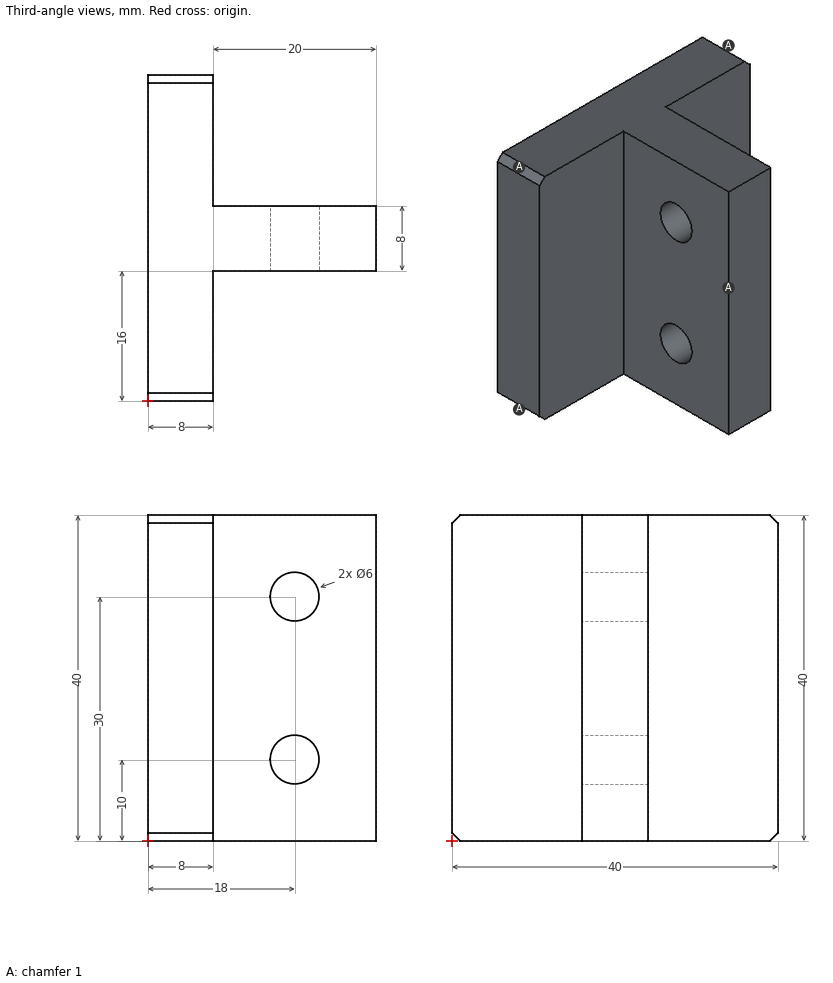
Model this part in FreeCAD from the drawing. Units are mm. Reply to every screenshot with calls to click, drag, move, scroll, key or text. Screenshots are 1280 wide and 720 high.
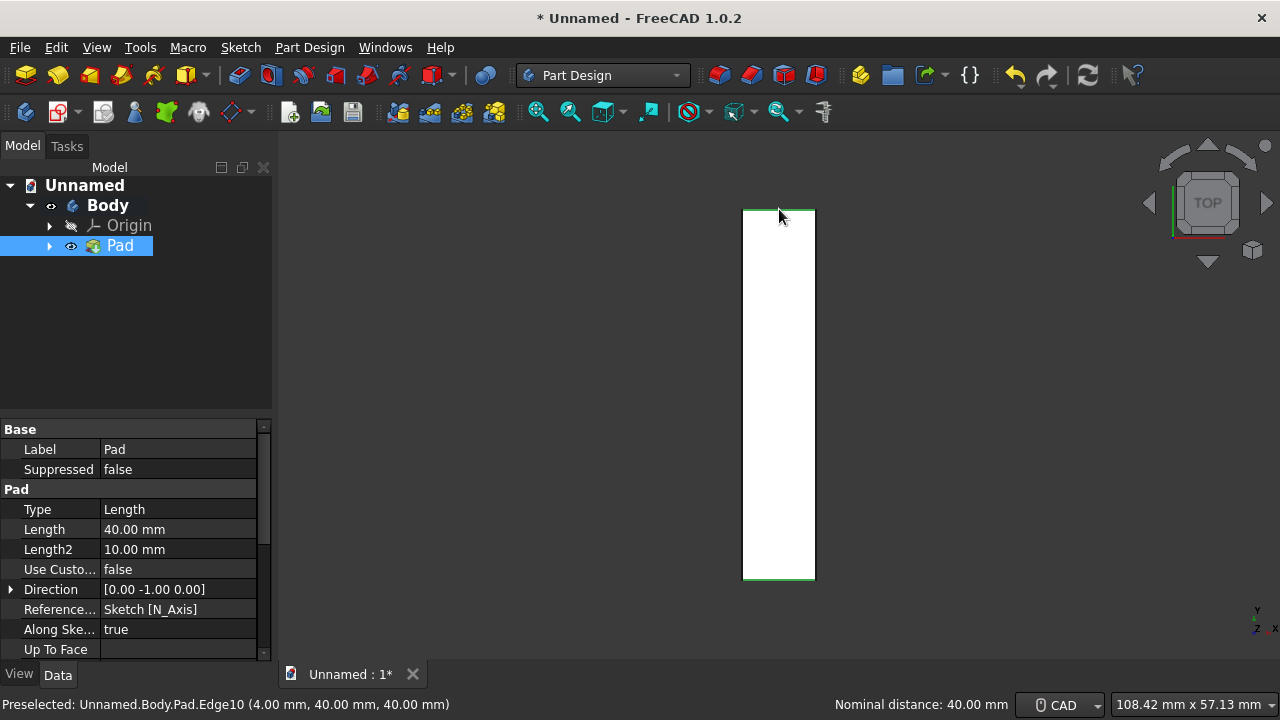
key(1)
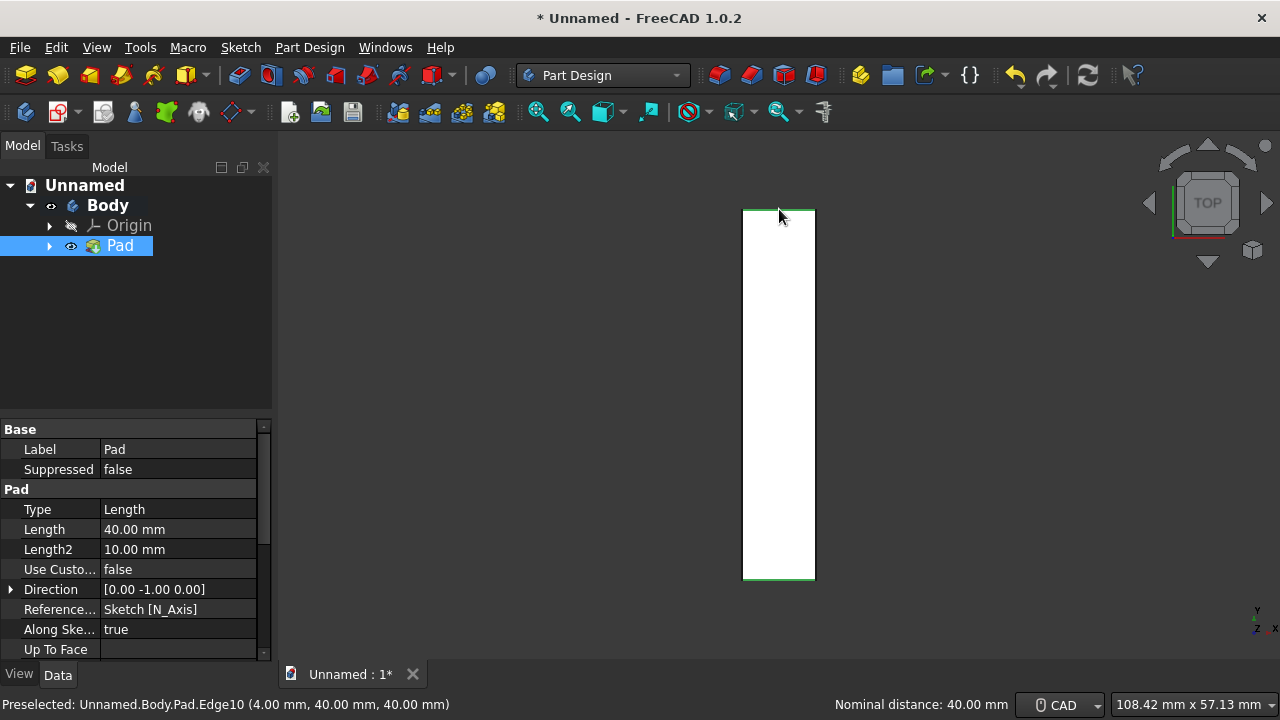
key(3)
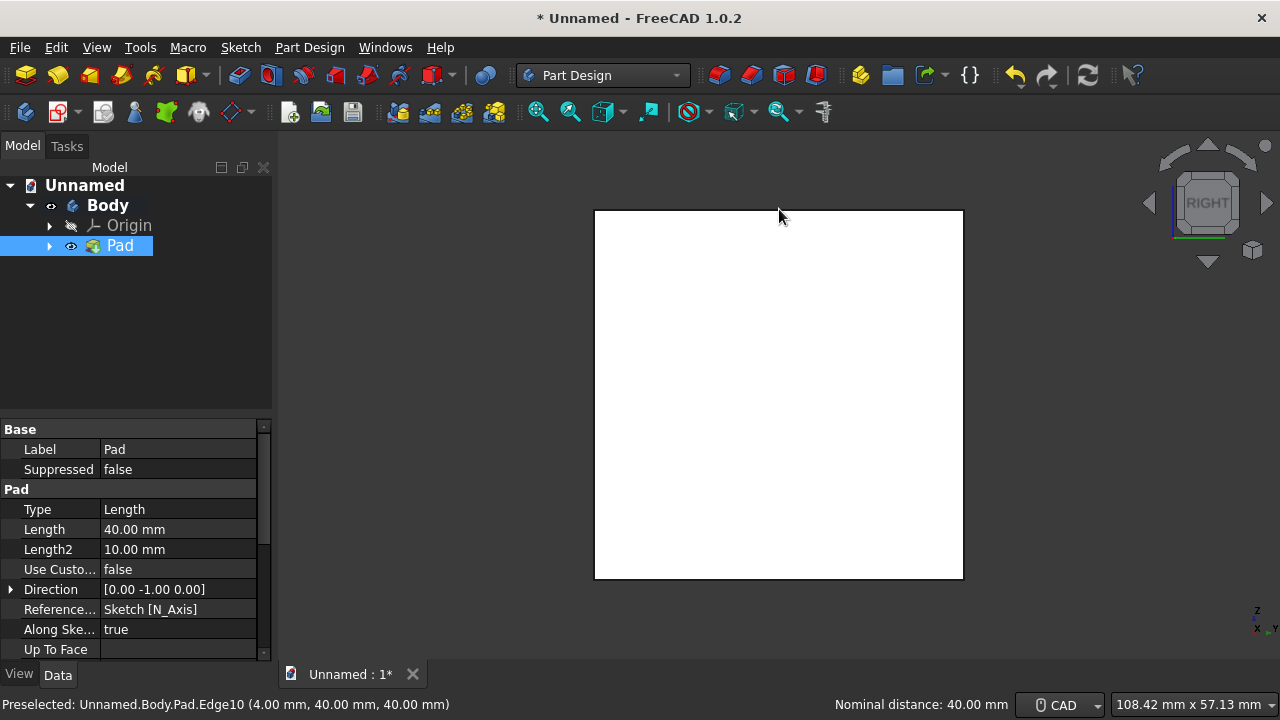
key(5)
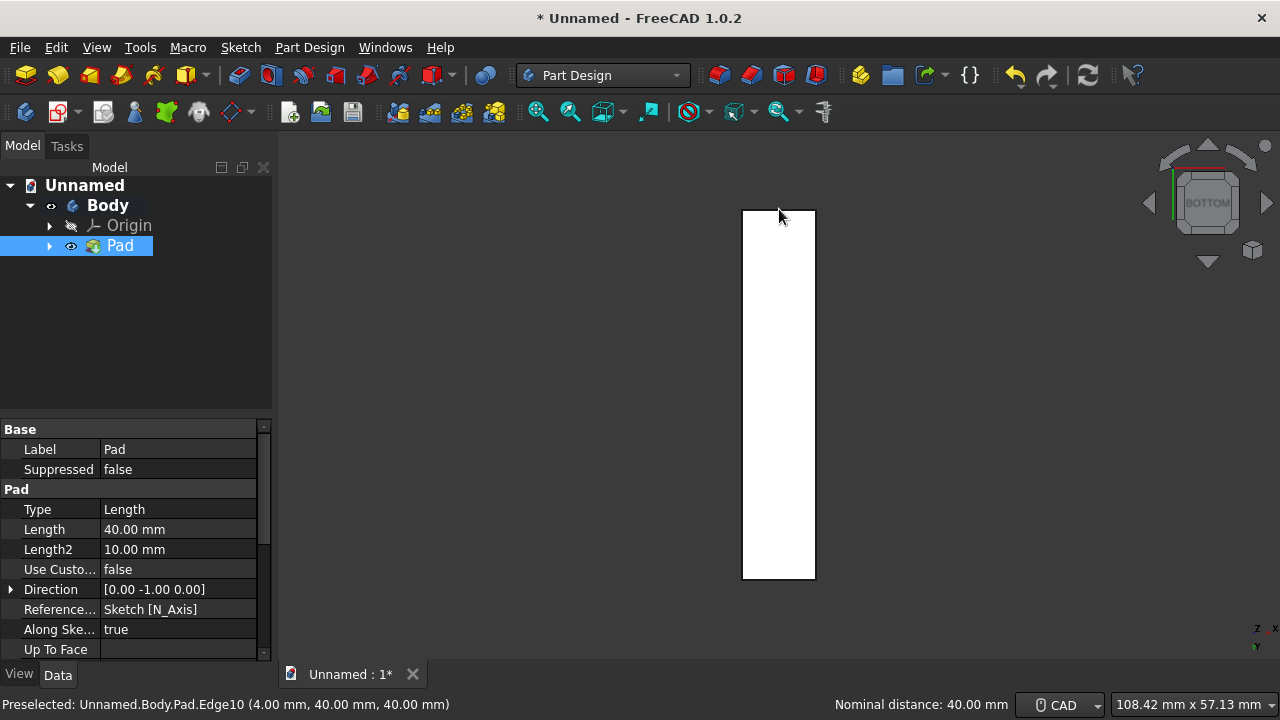
click(779, 209, ctrl)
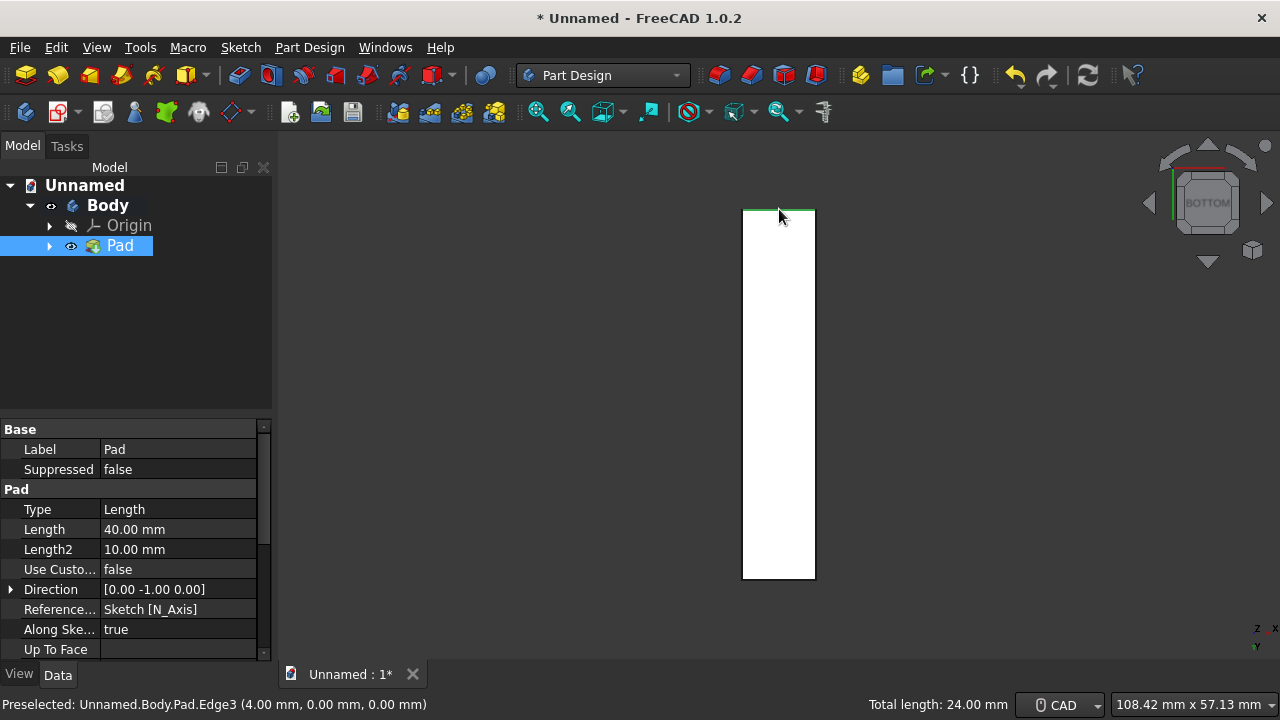
key(4)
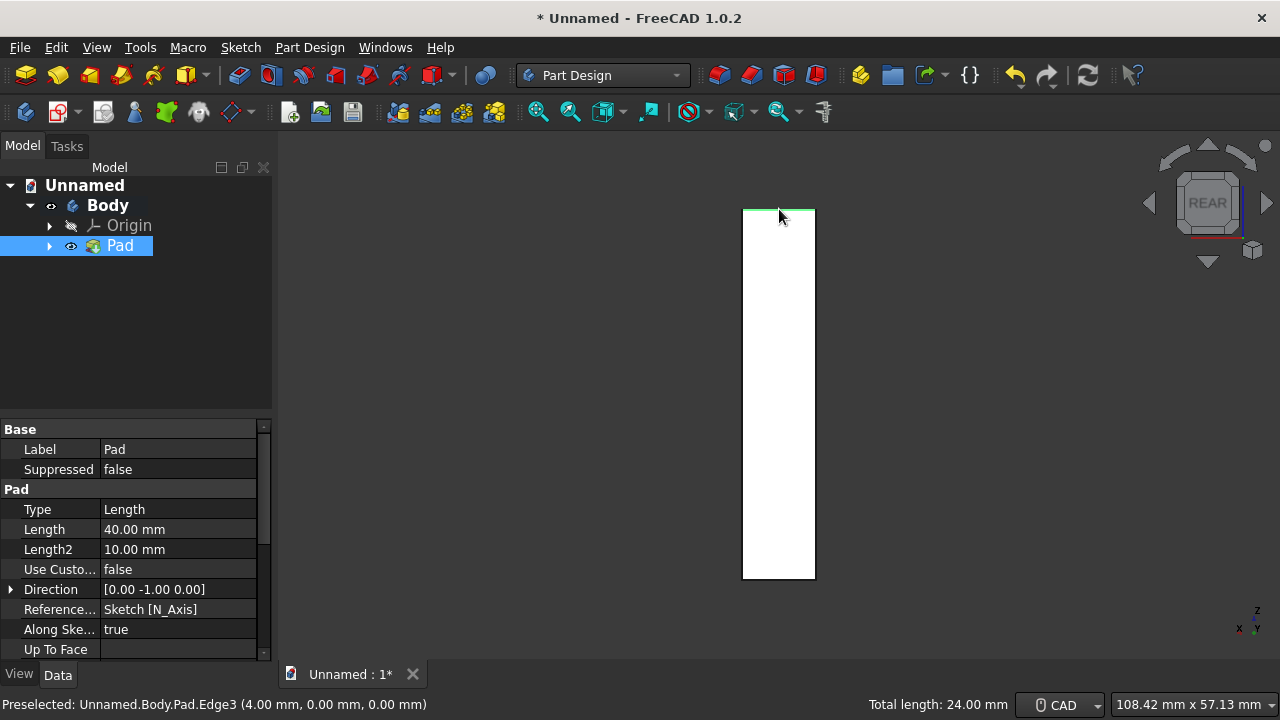
click(779, 579, ctrl)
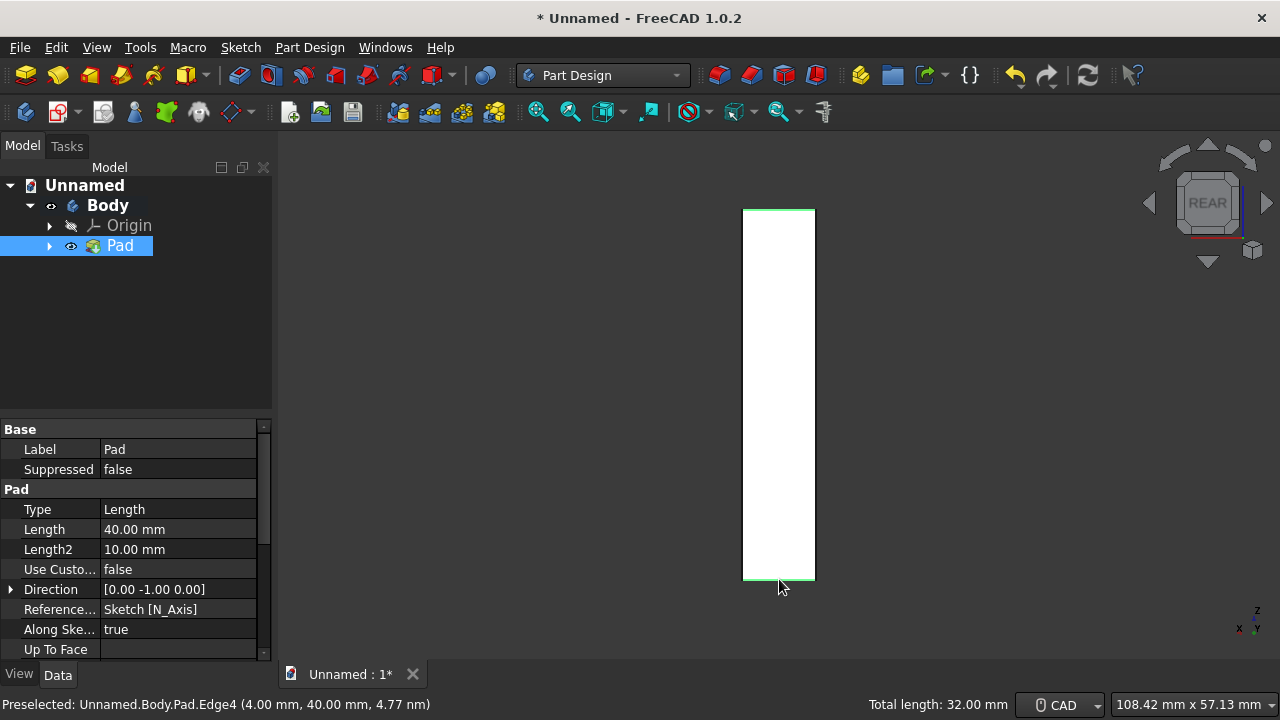
click(752, 76)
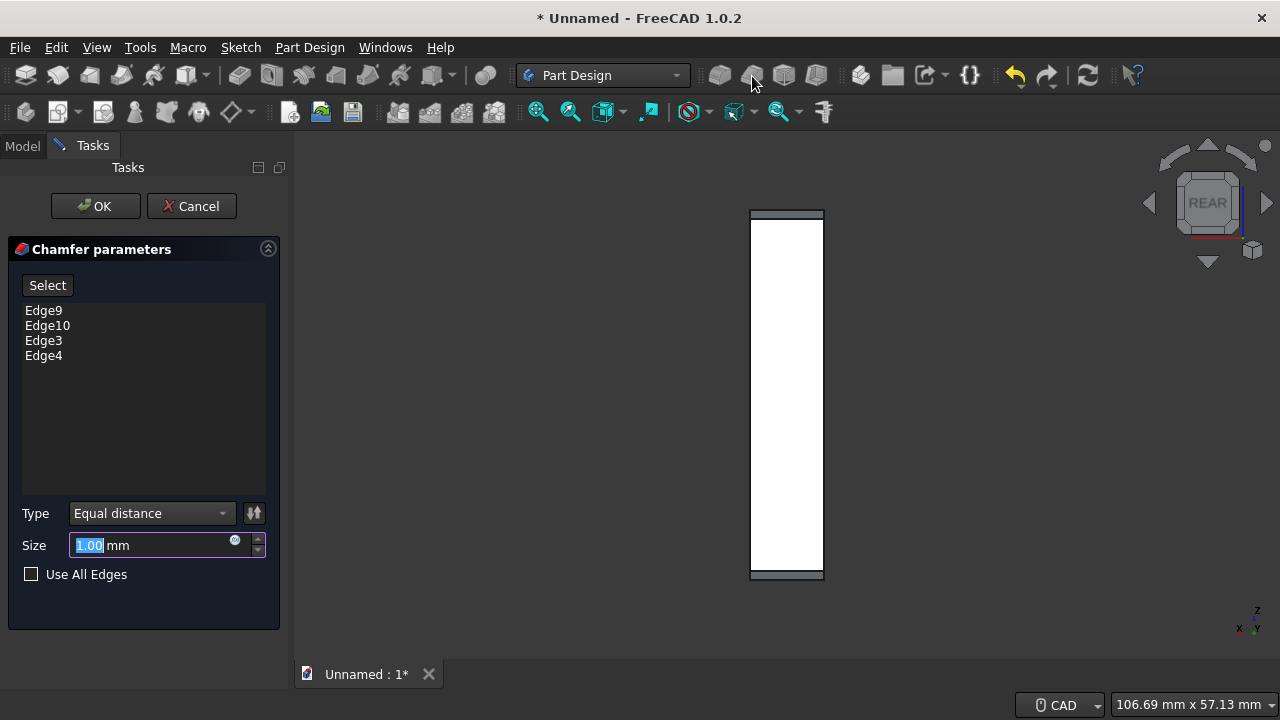
text(1)
key(Tab)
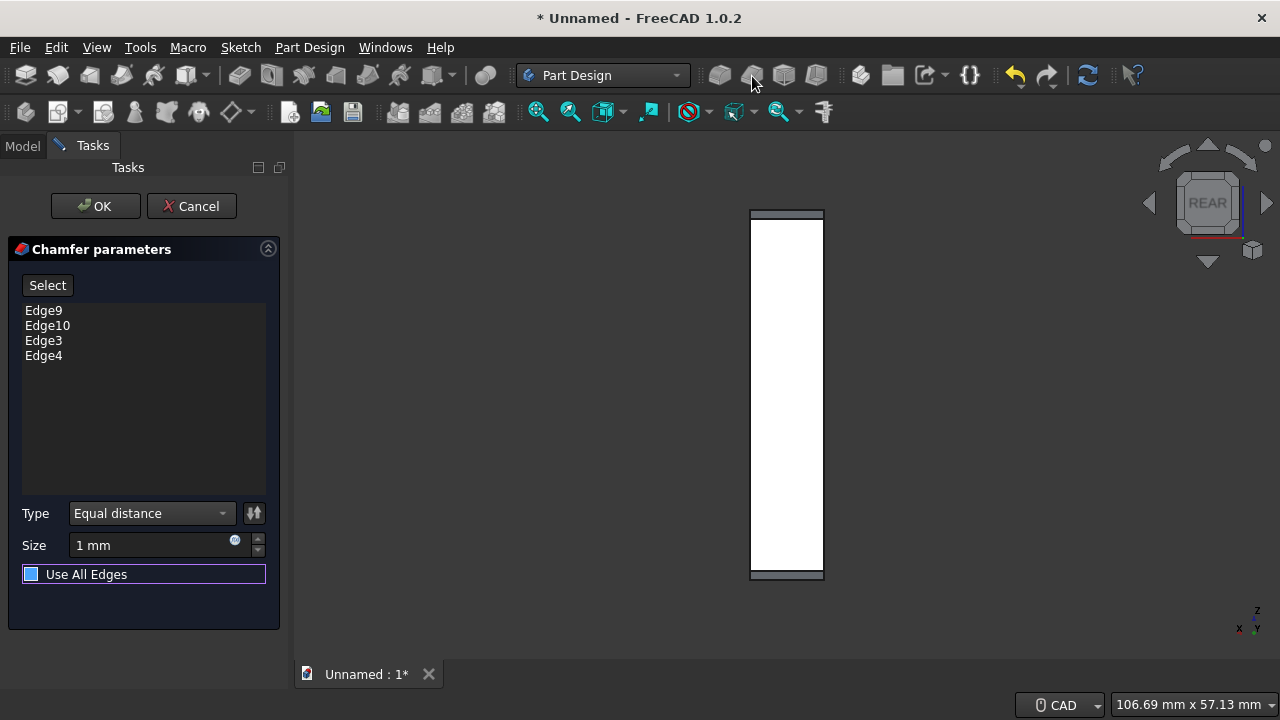
click(96, 206)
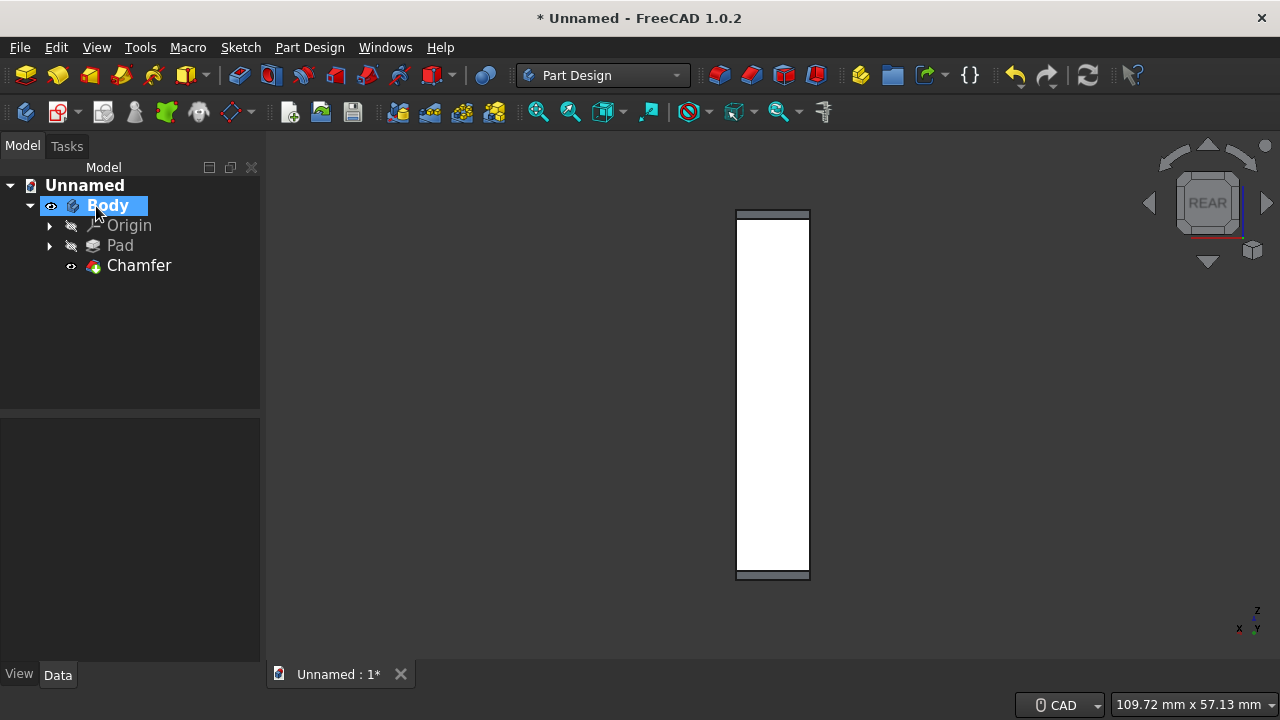
key(0)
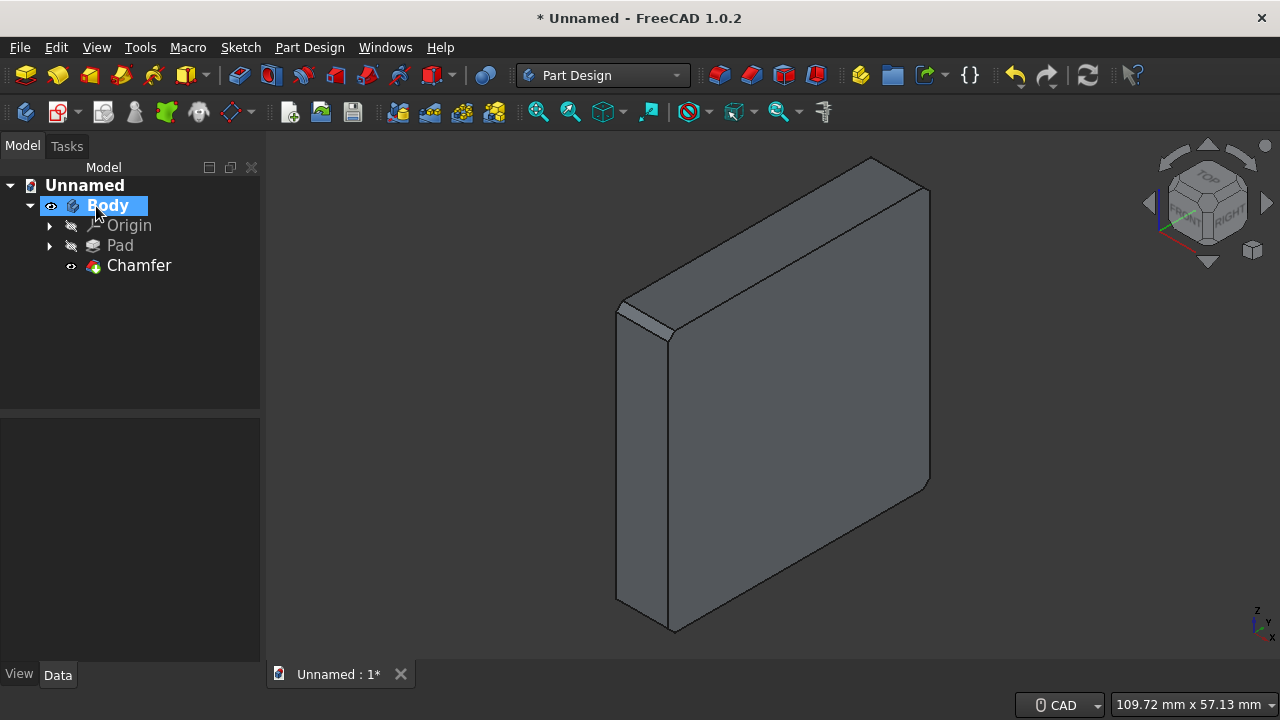
click(844, 202)